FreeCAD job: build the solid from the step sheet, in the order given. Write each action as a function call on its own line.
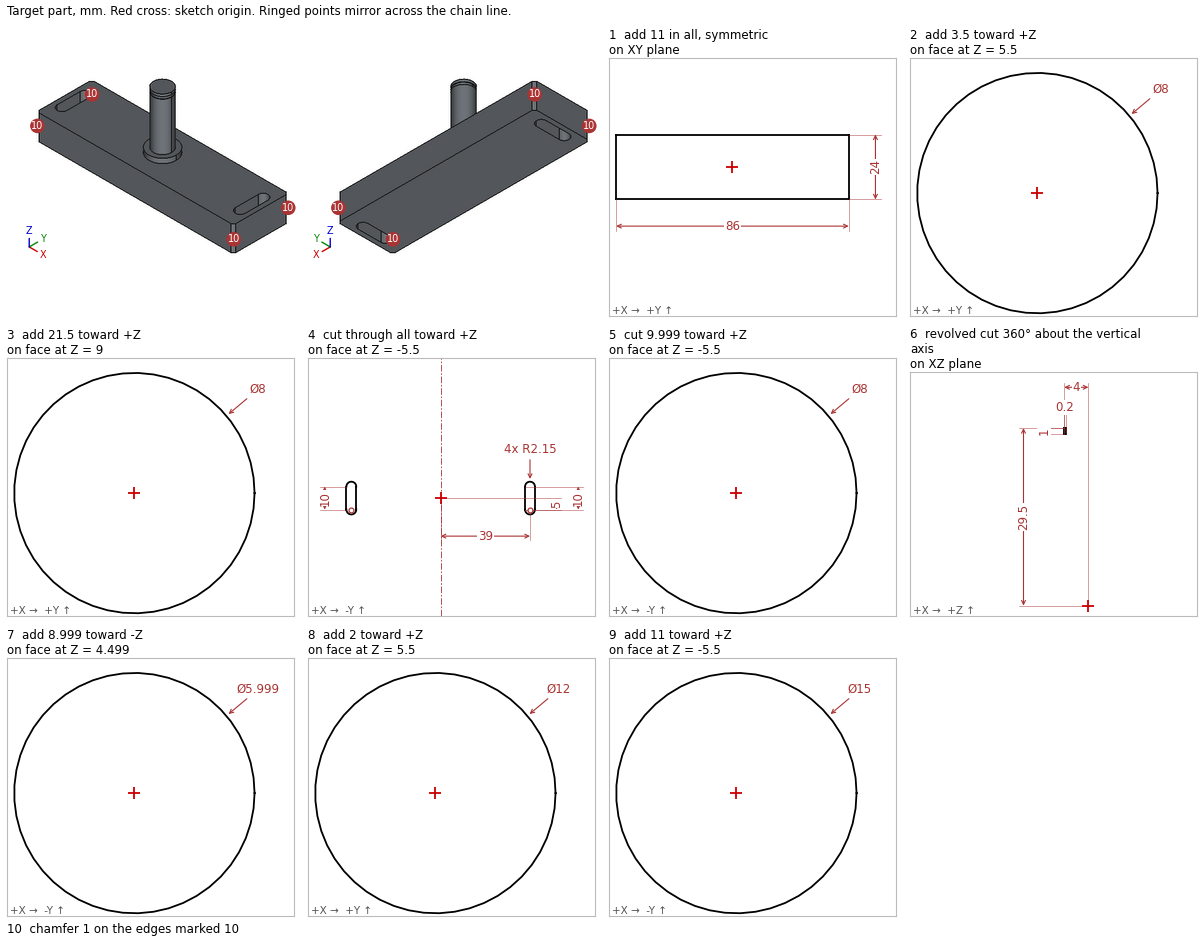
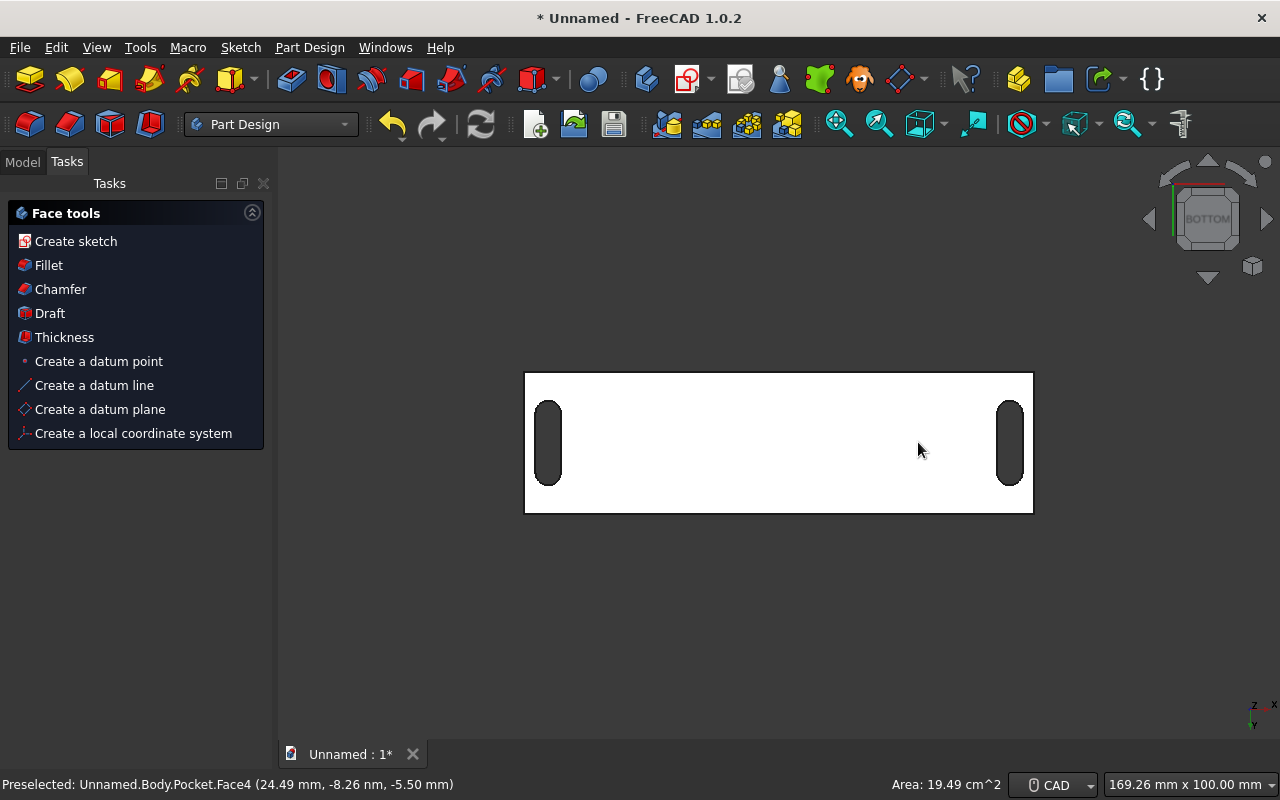
click(688, 80)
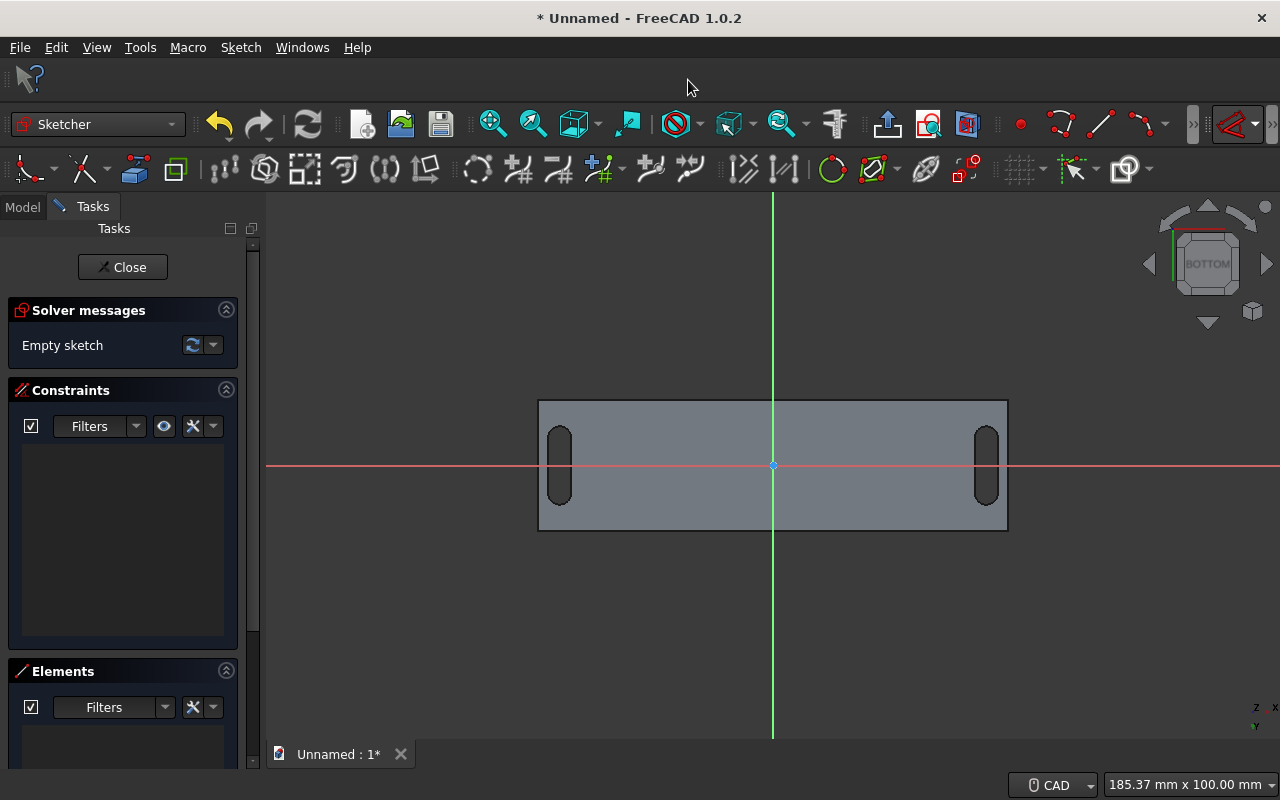
scroll(784, 466, up, 10)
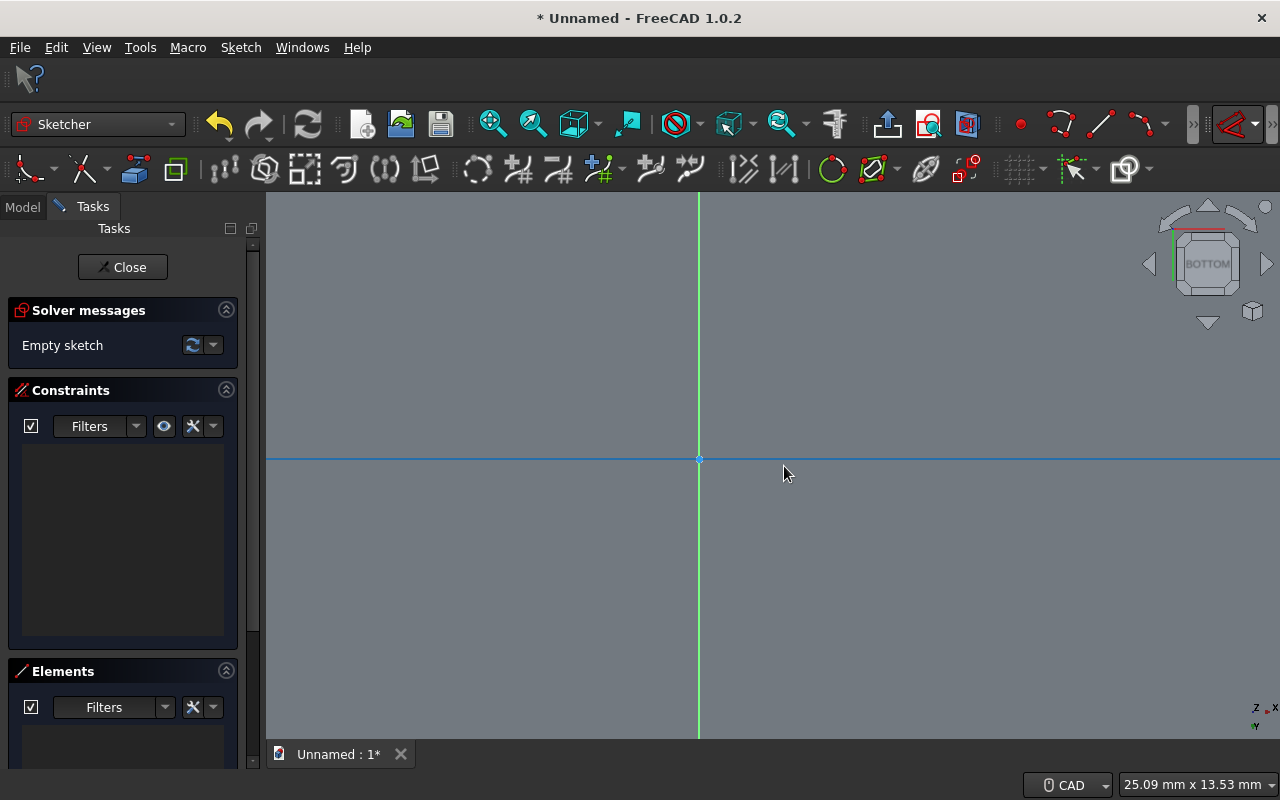
key(g)
key(c)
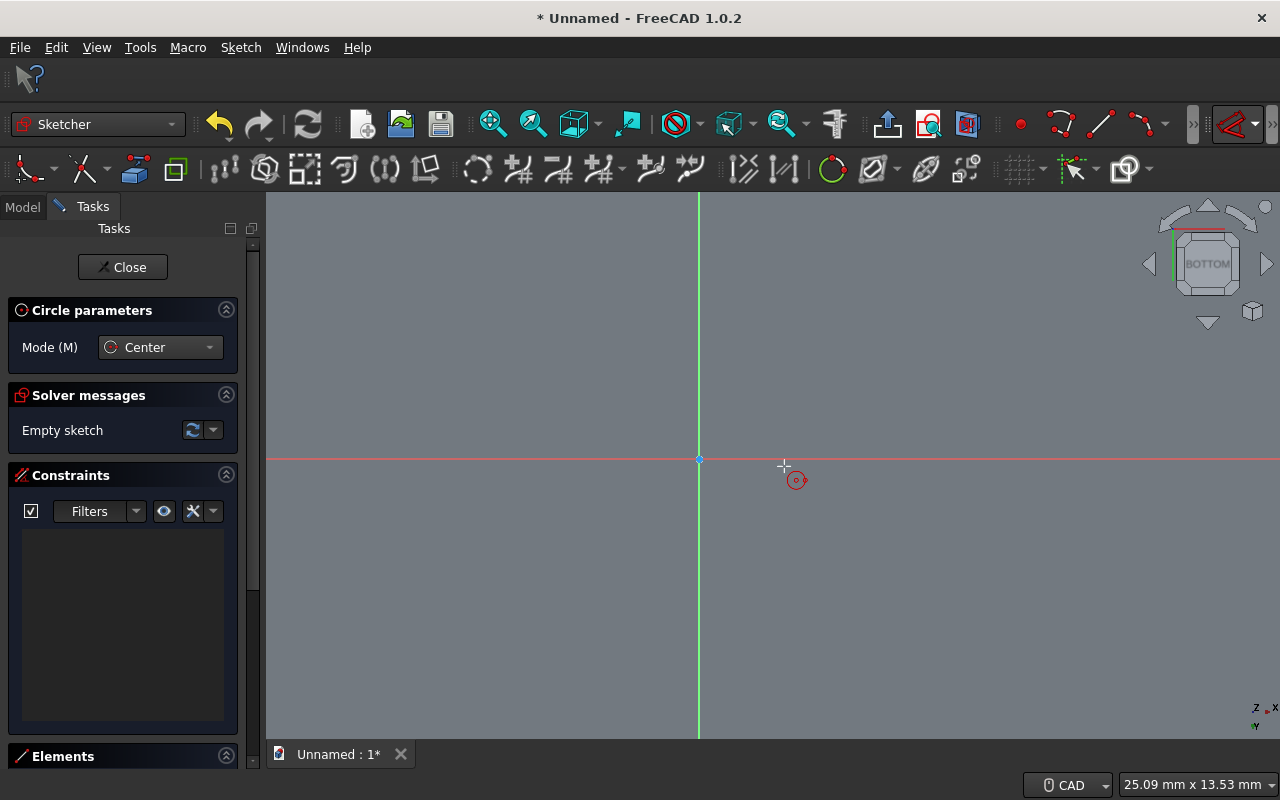
click(699, 459)
move(814, 345)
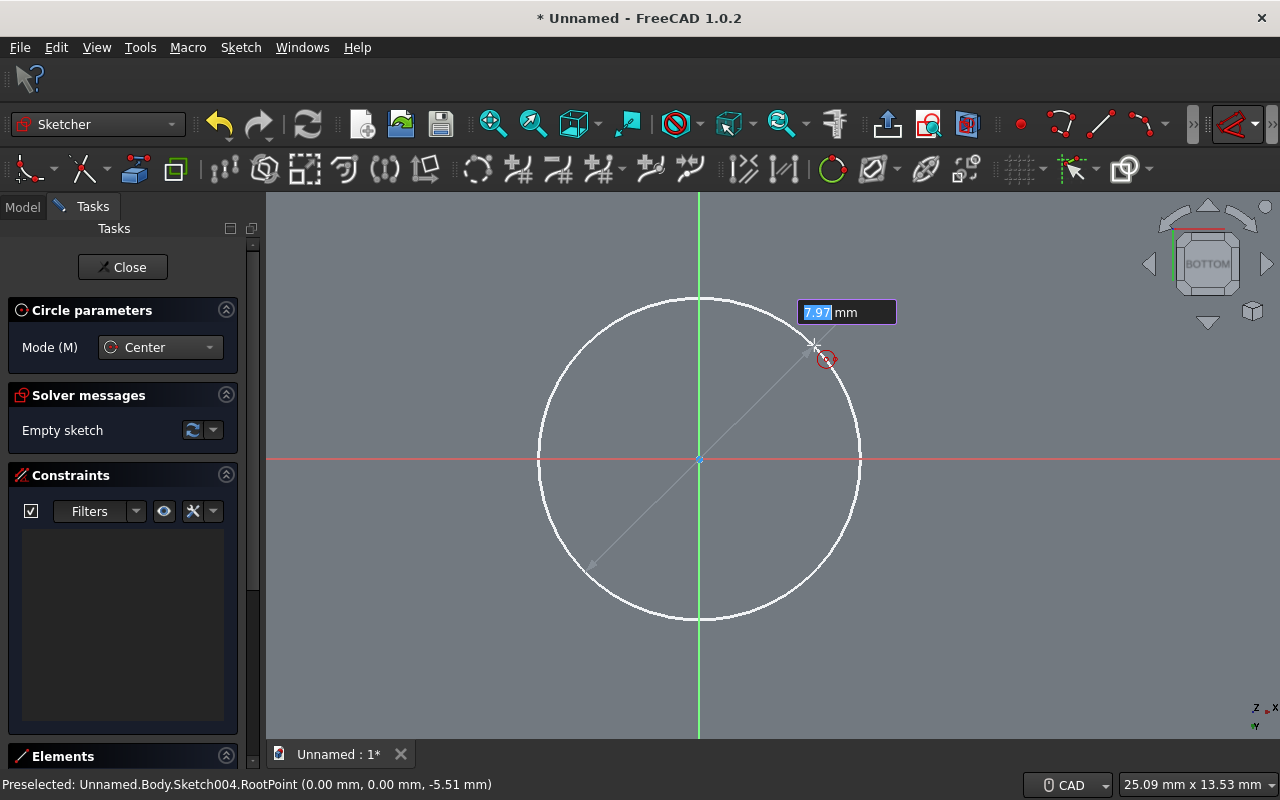
text(8)
key(Return)
key(Escape)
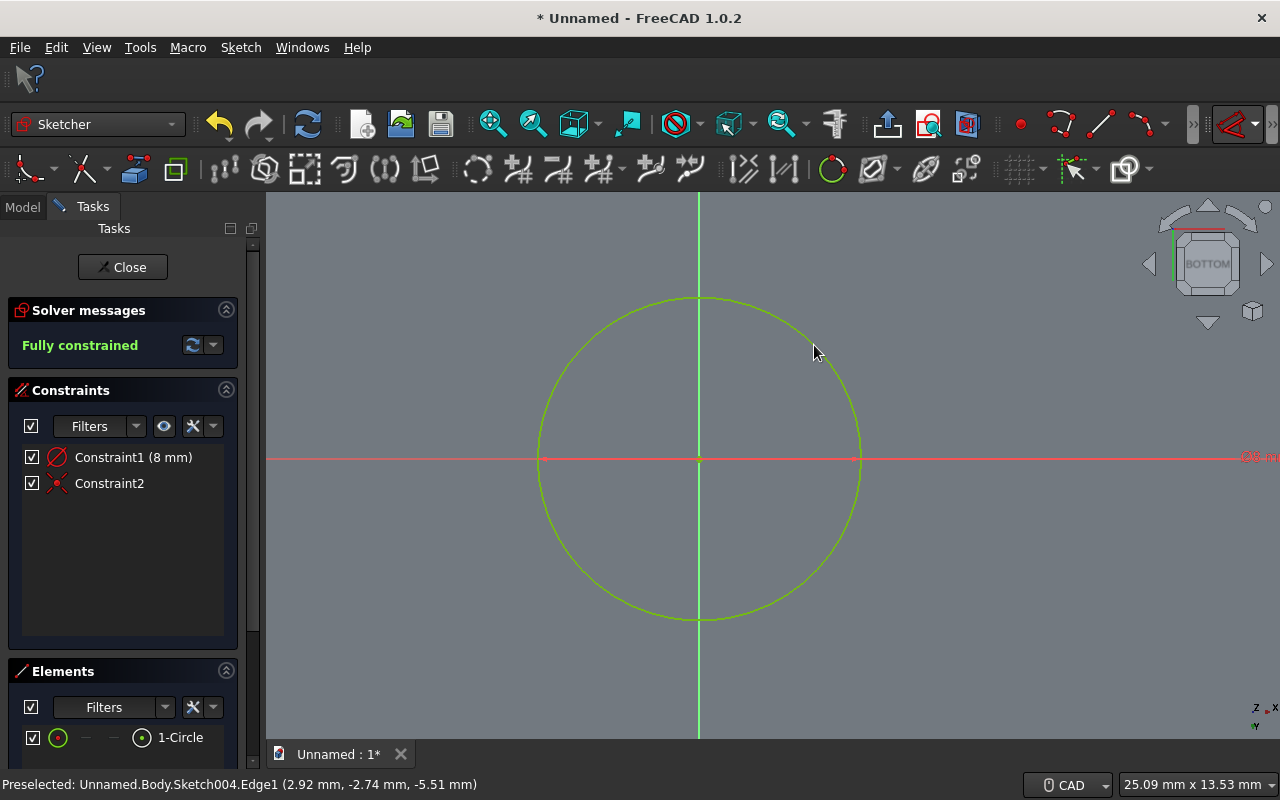
click(123, 267)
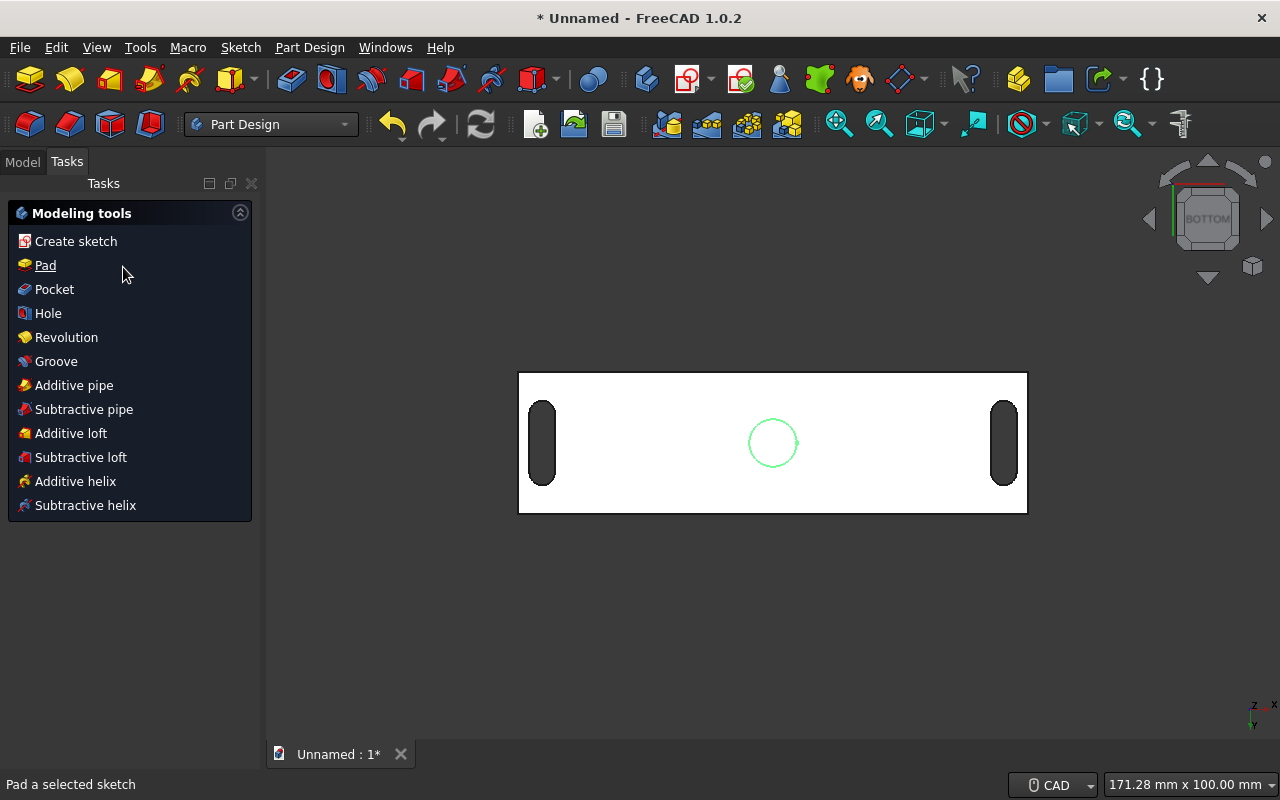
click(292, 80)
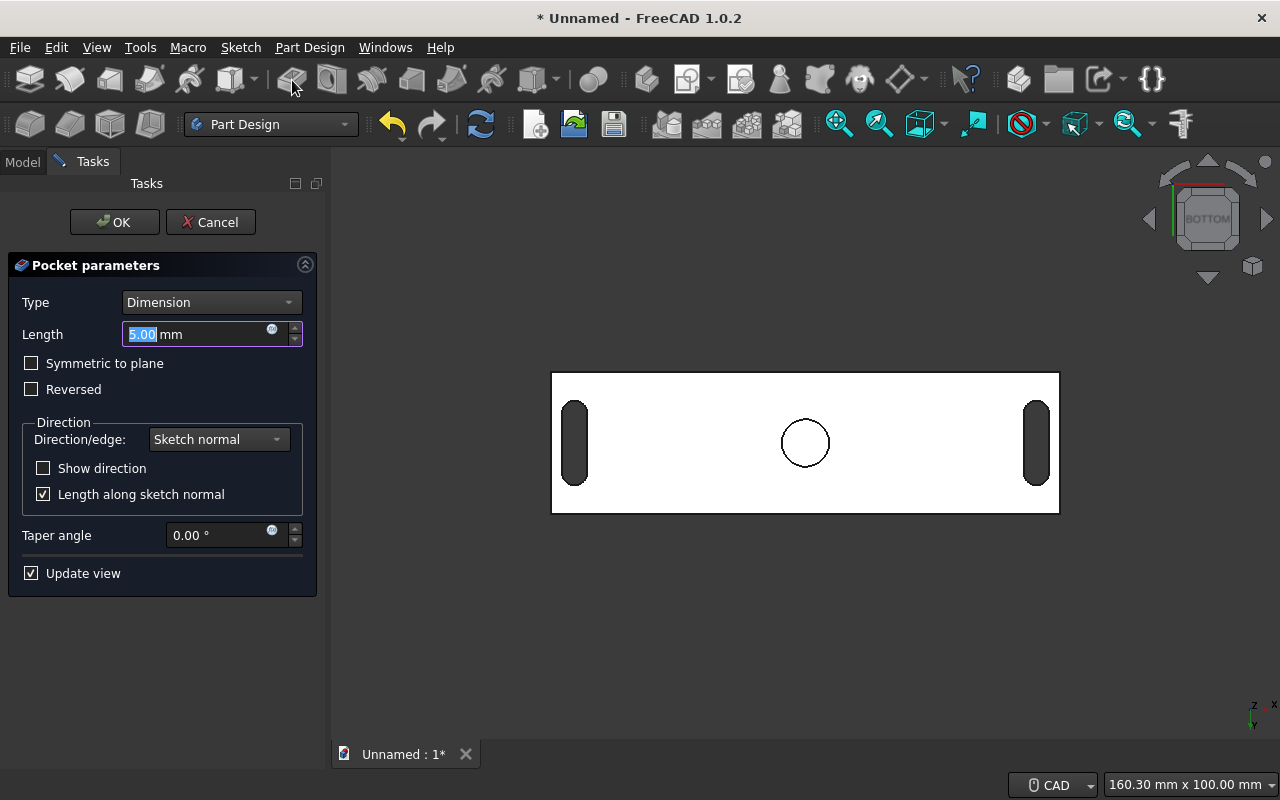
text(9.999)
key(Tab)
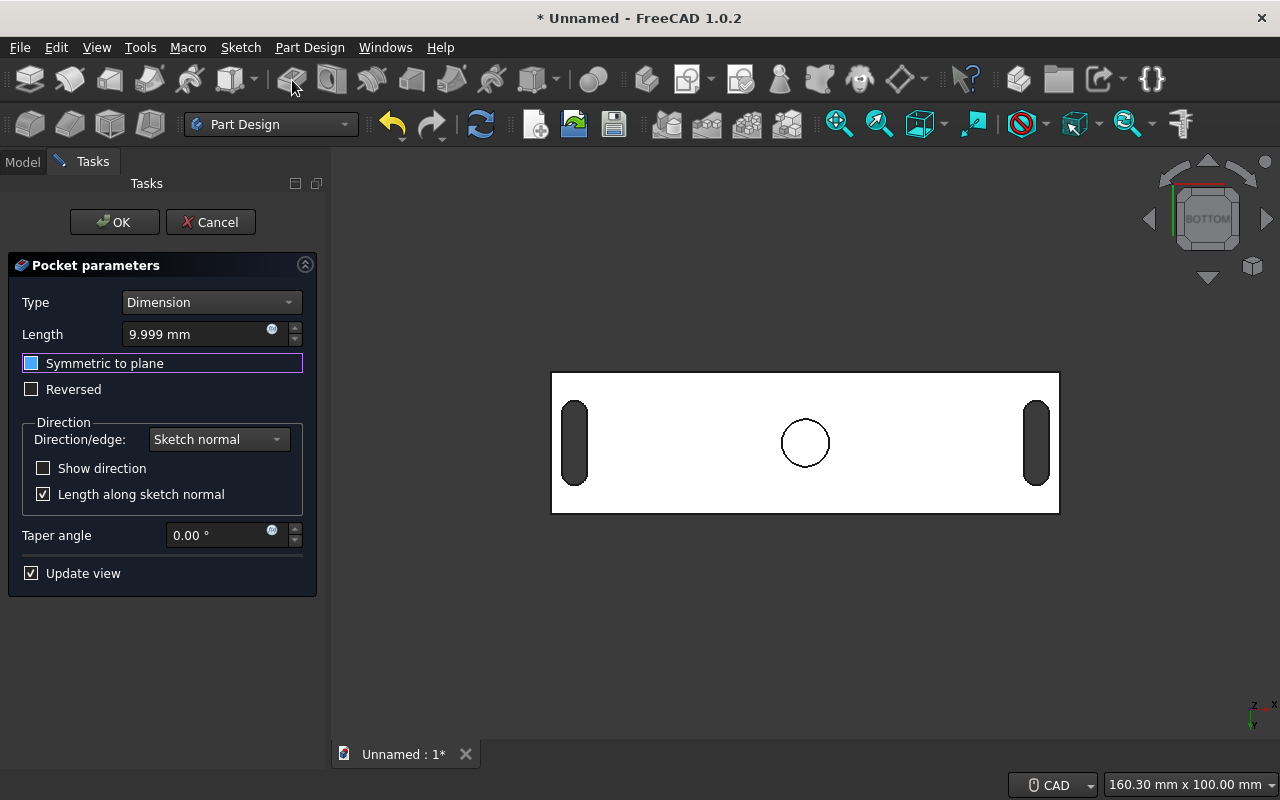
click(115, 222)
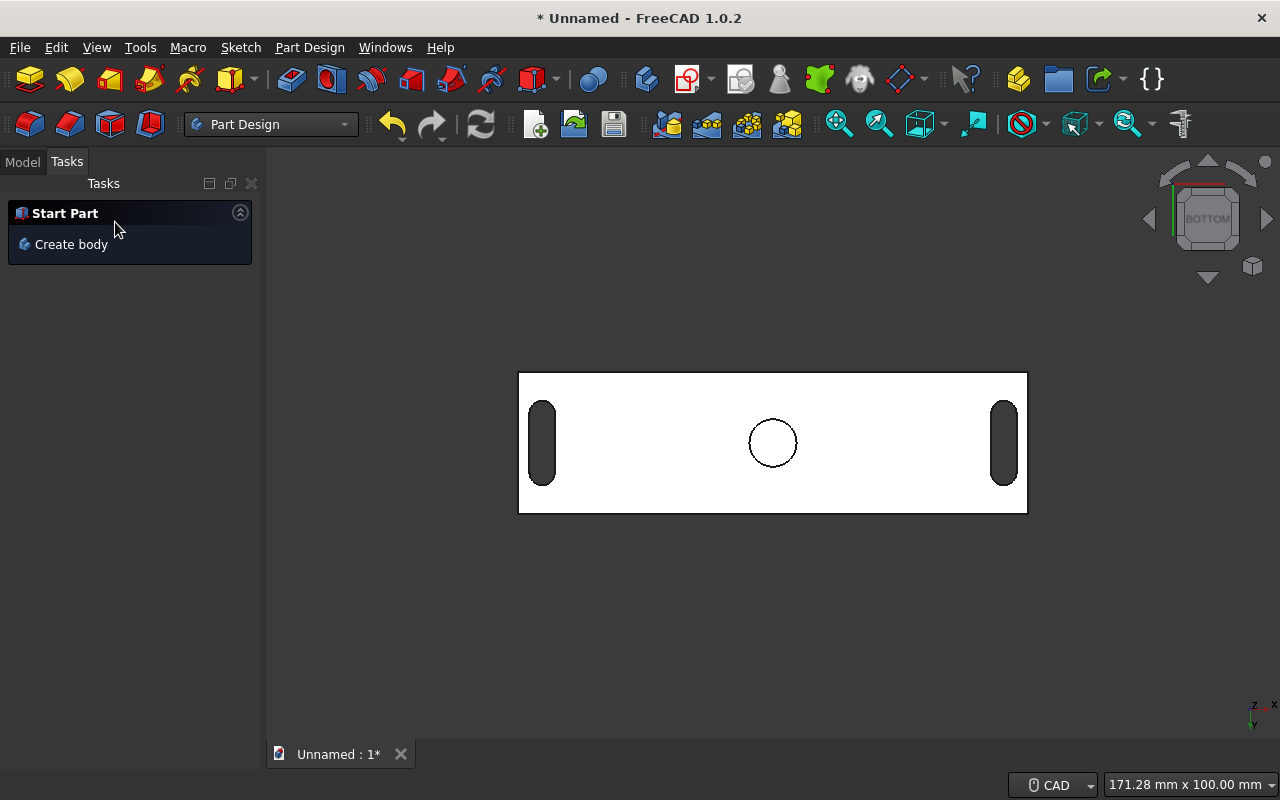
click(688, 80)